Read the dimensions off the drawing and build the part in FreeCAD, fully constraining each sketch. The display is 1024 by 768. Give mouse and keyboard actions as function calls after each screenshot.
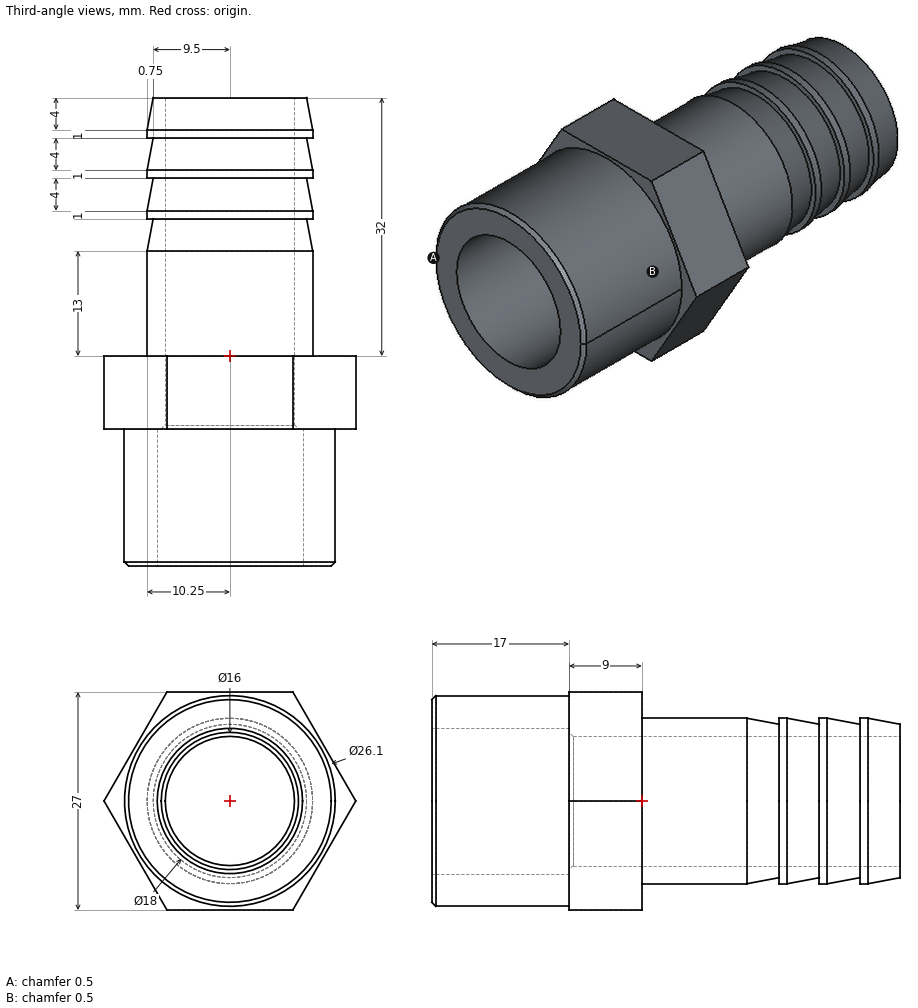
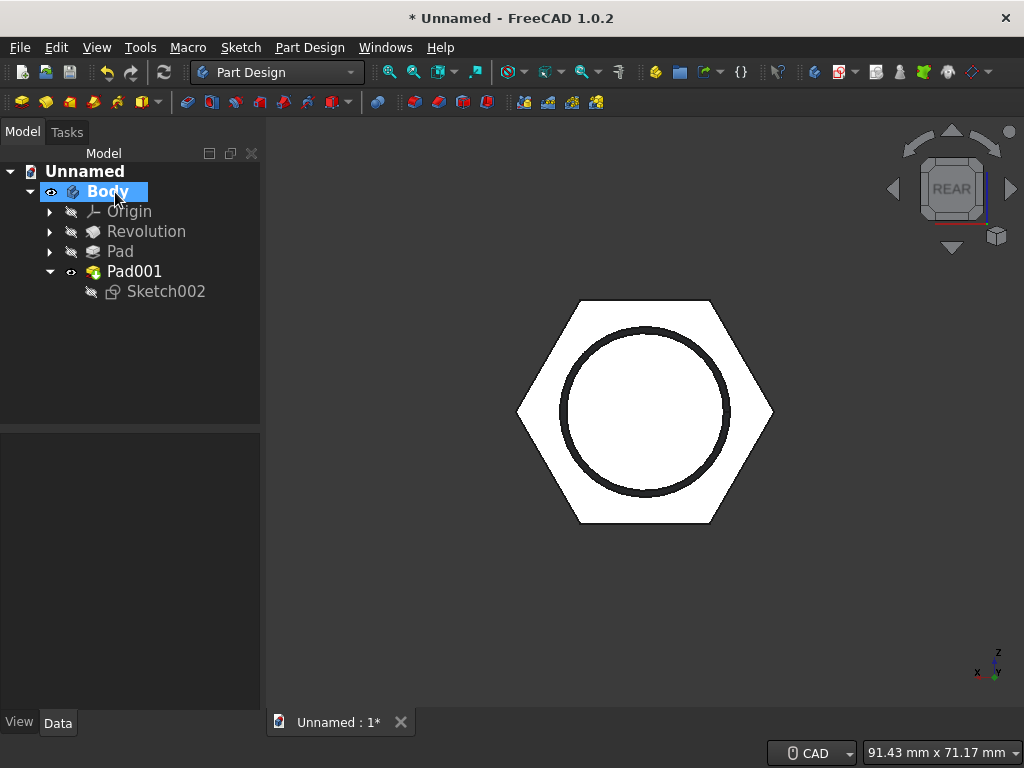
key(v)
key(f)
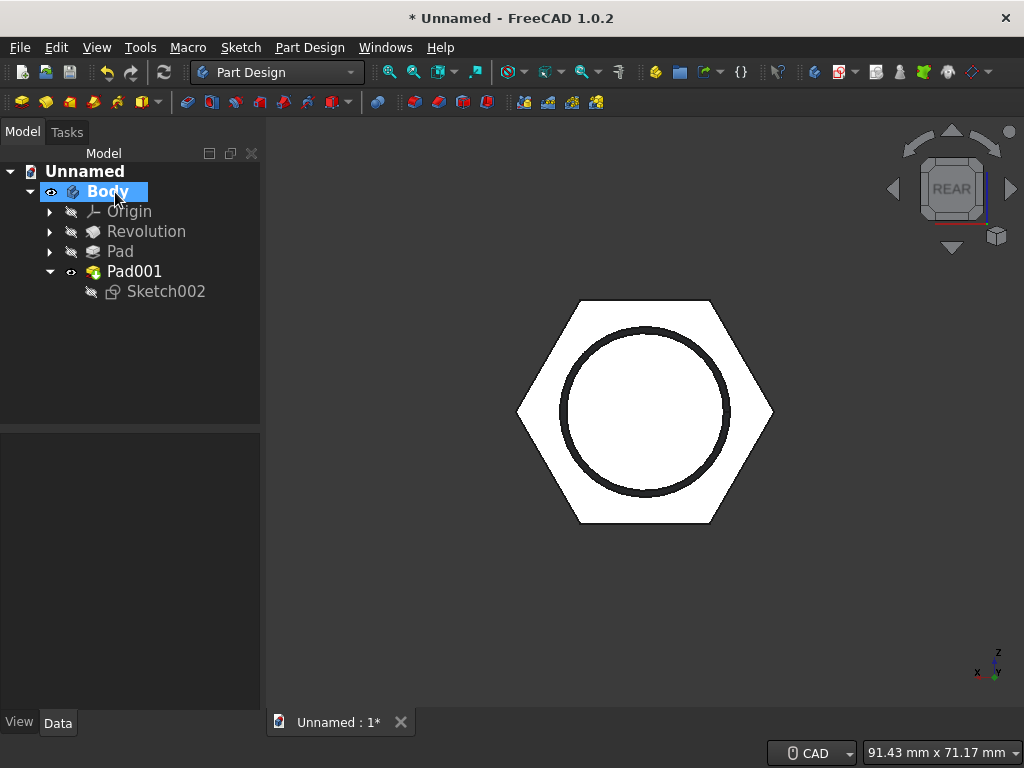
click(645, 411)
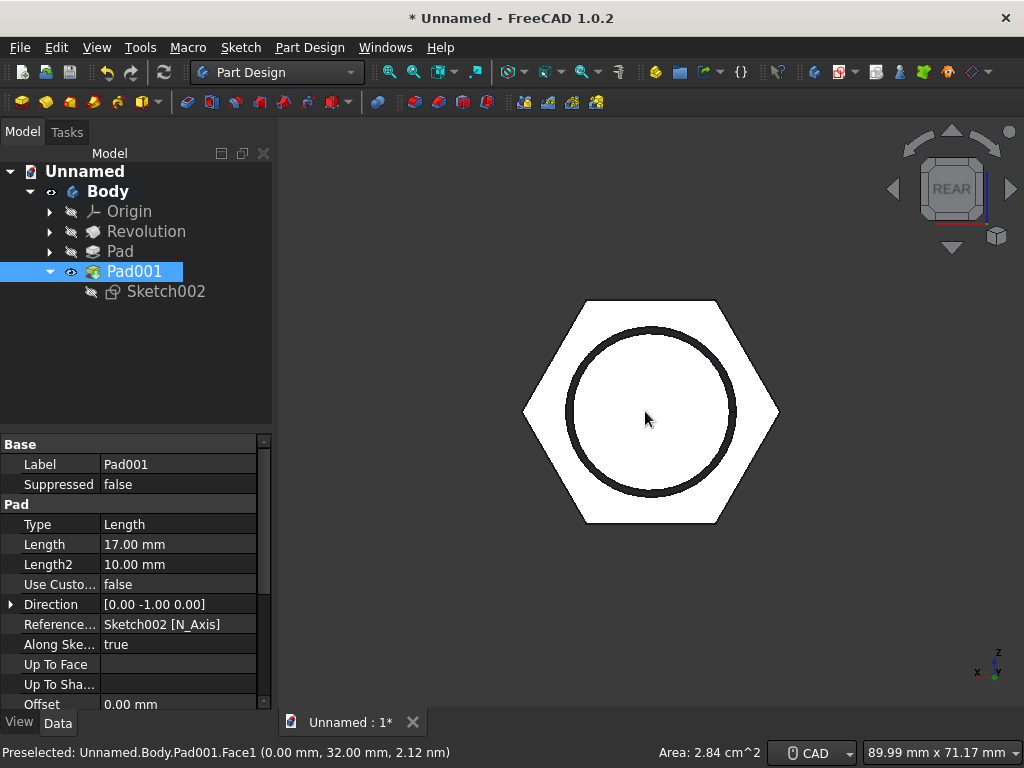
click(840, 72)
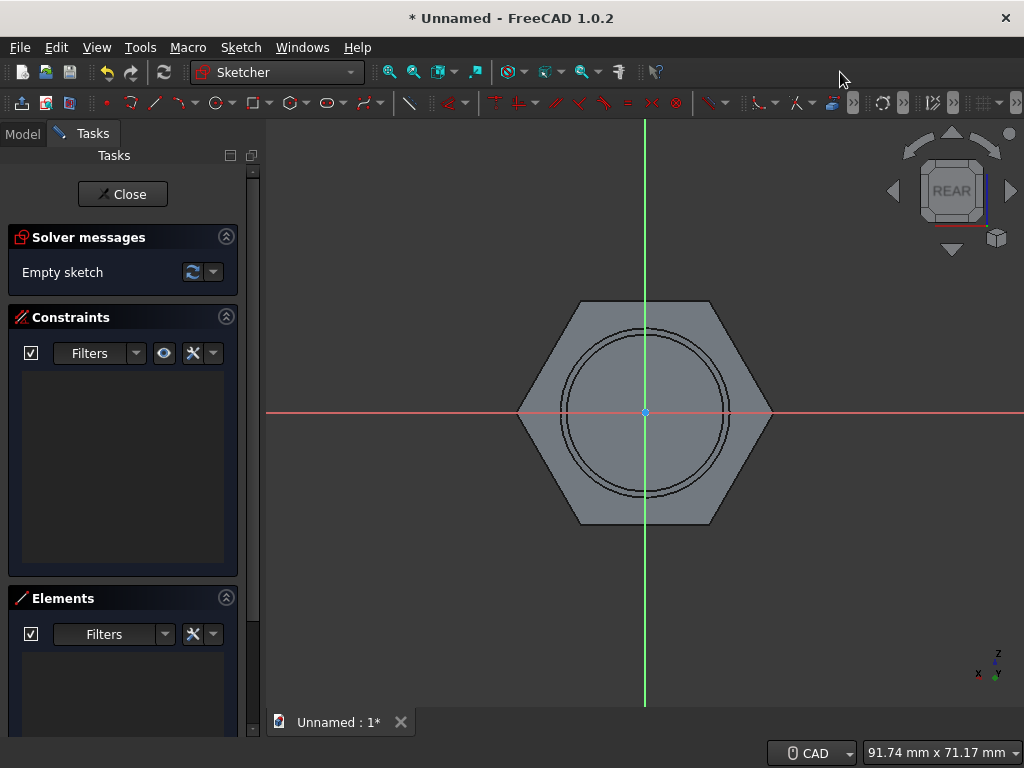
scroll(685, 413, up, 5)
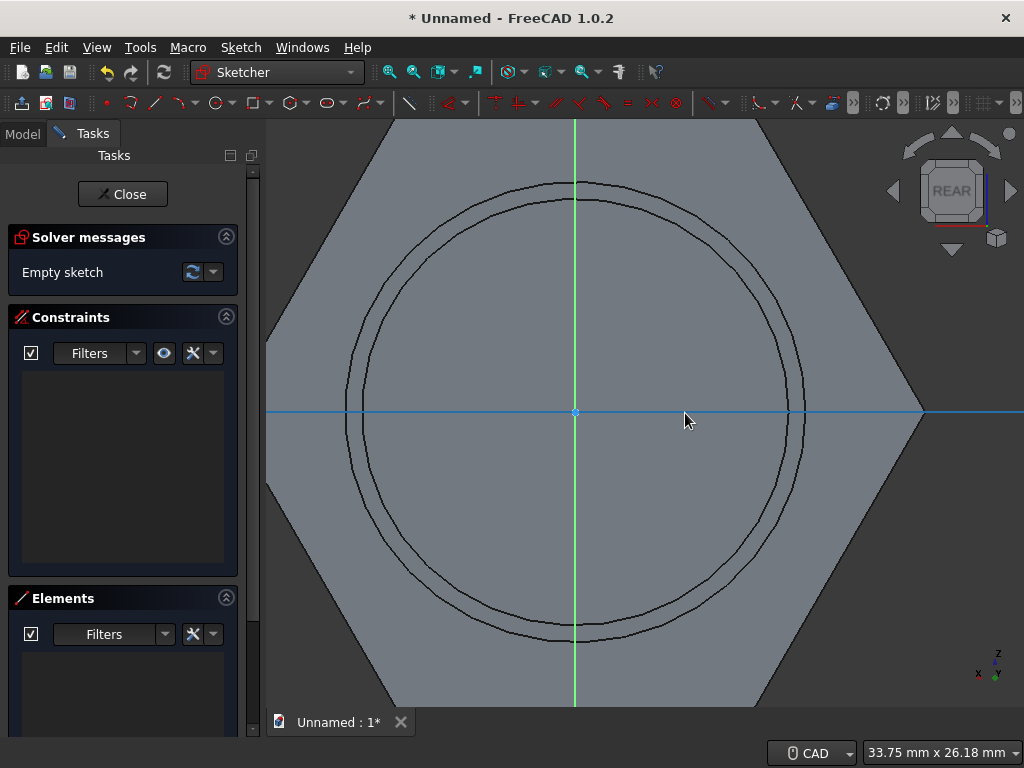
key(g)
key(c)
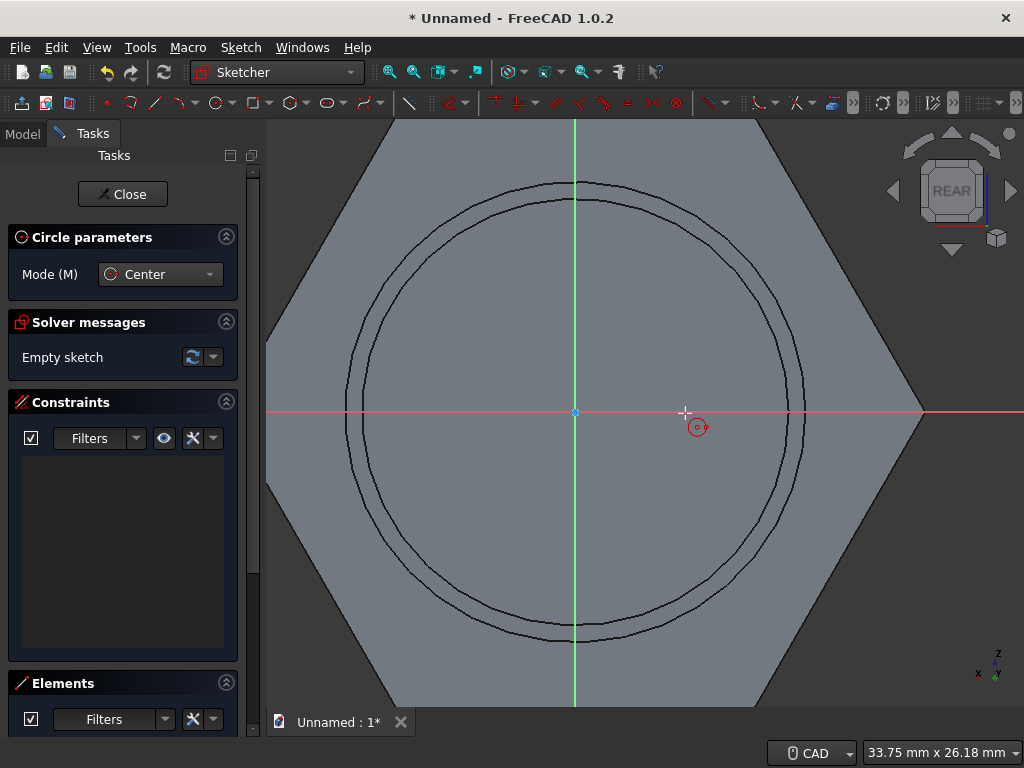
click(575, 412)
click(702, 285)
key(Escape)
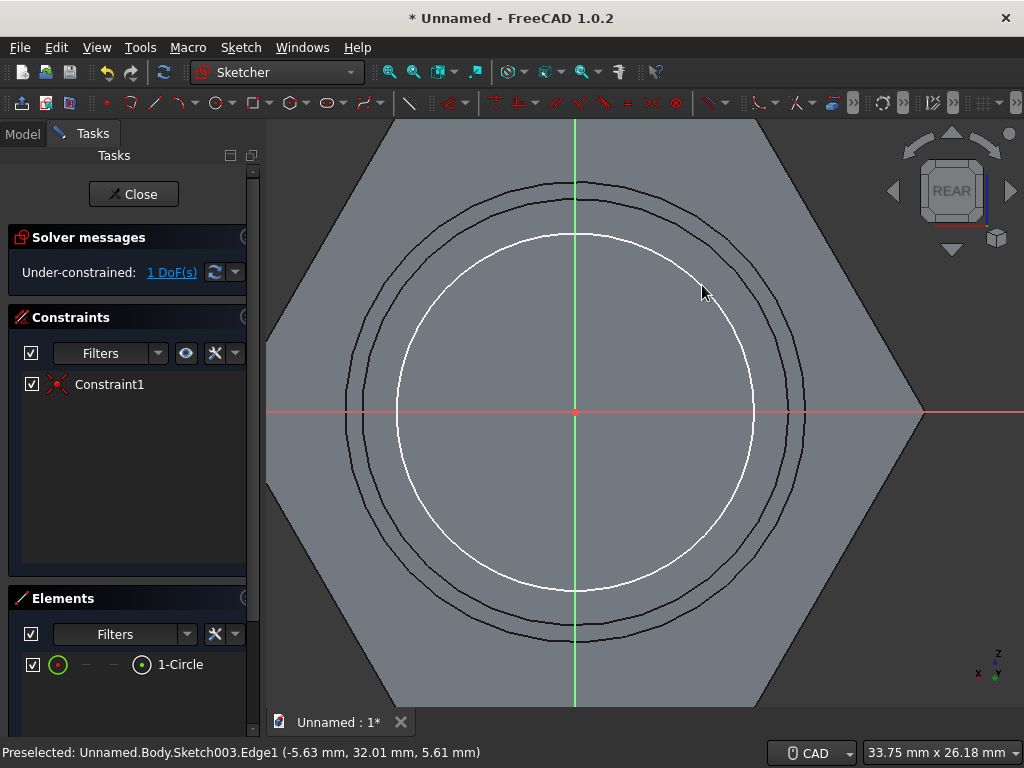
key(d)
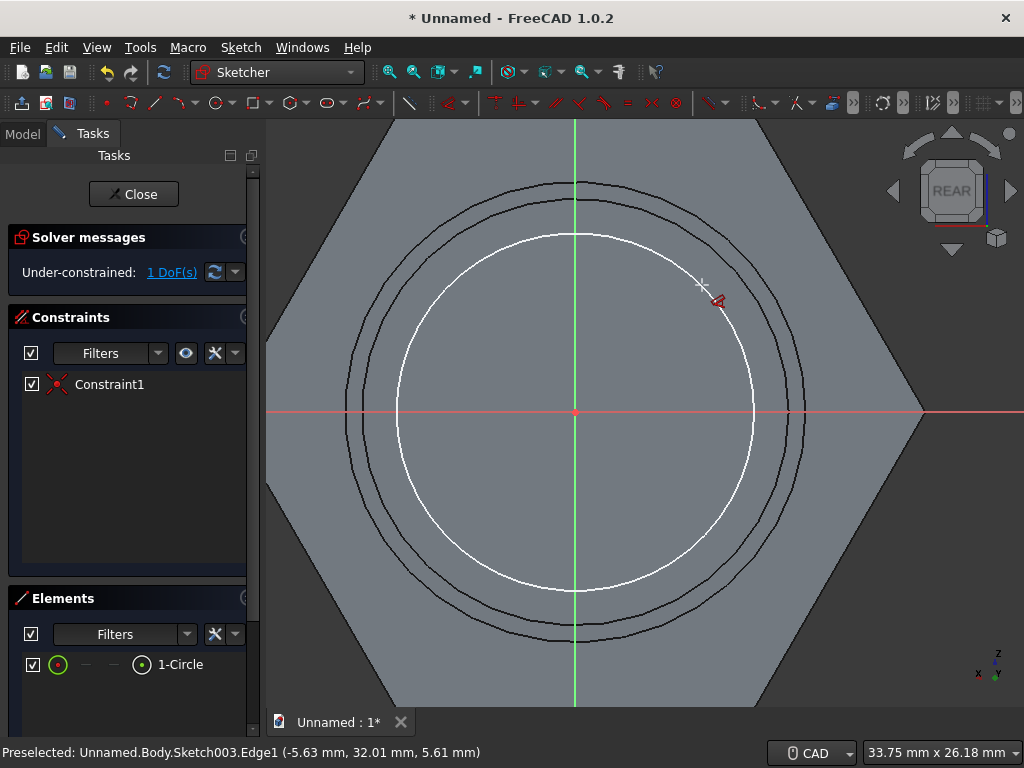
click(701, 285)
click(723, 262)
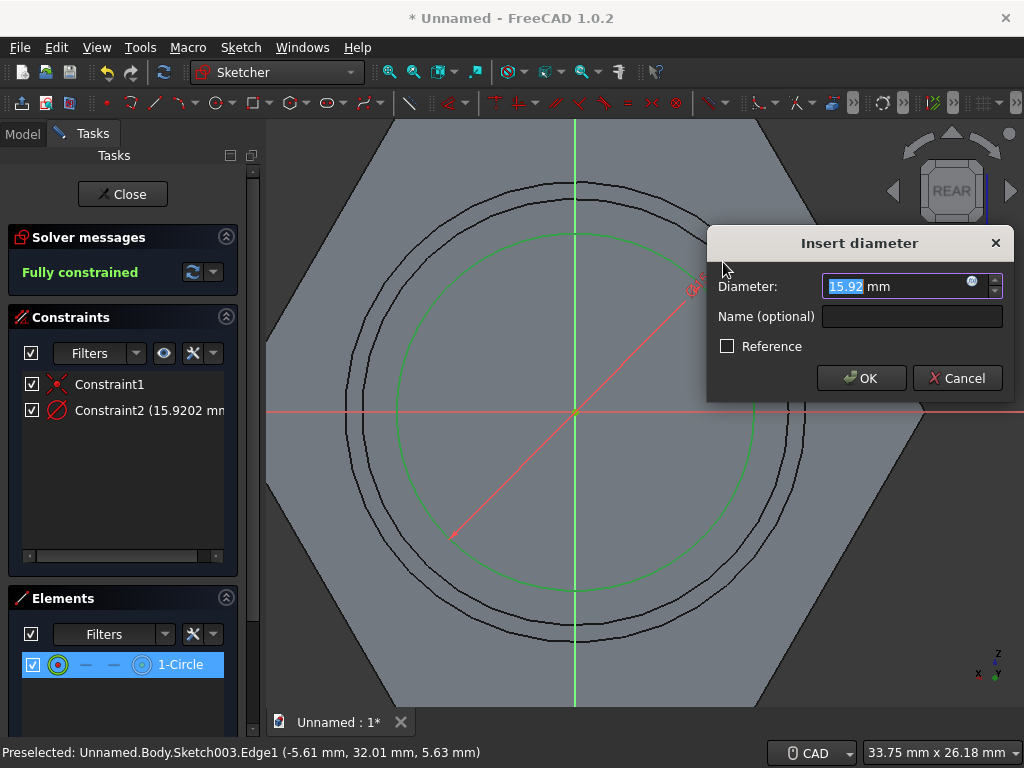
text(16)
key(Return)
key(Escape)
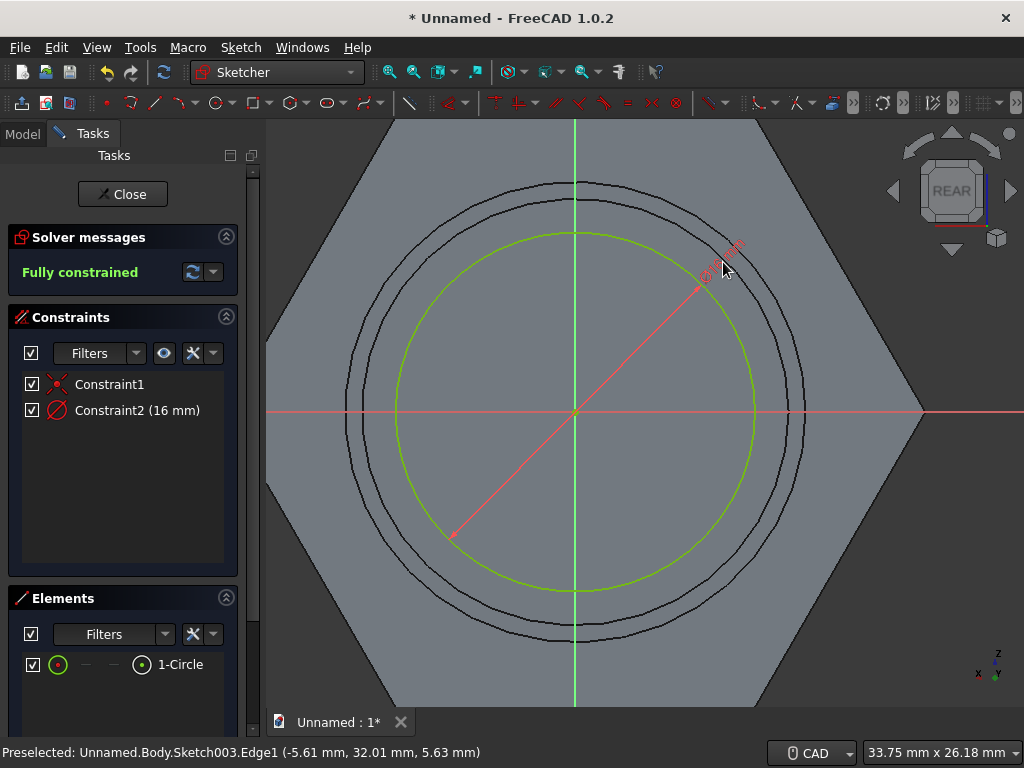
click(123, 194)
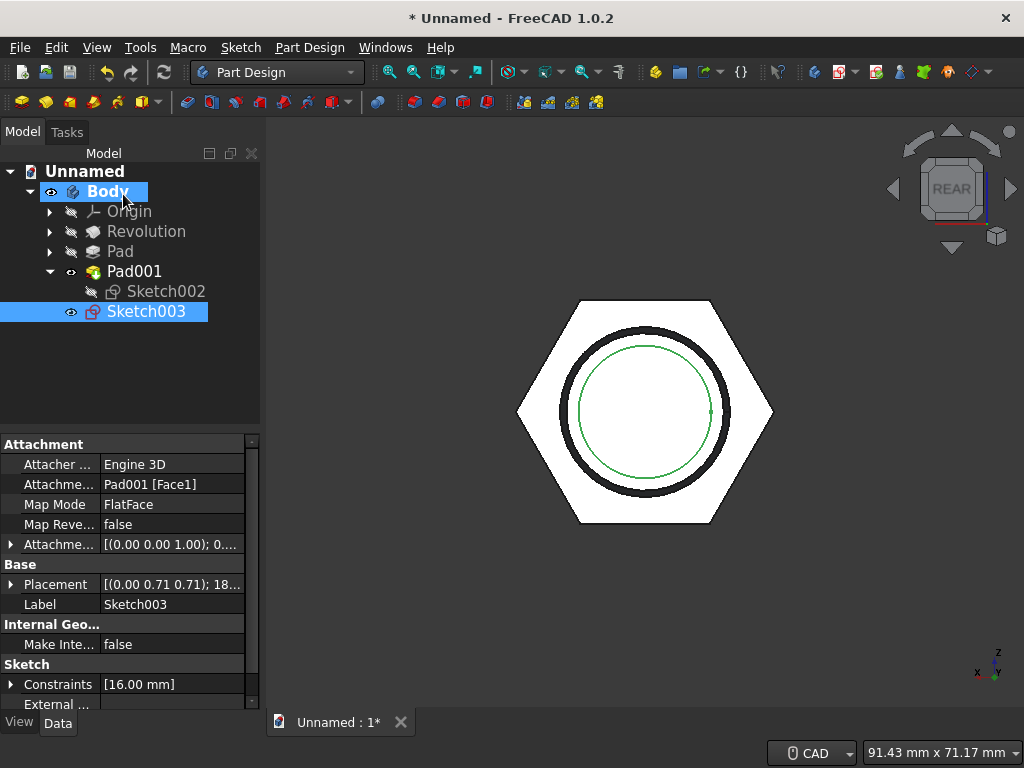
click(188, 102)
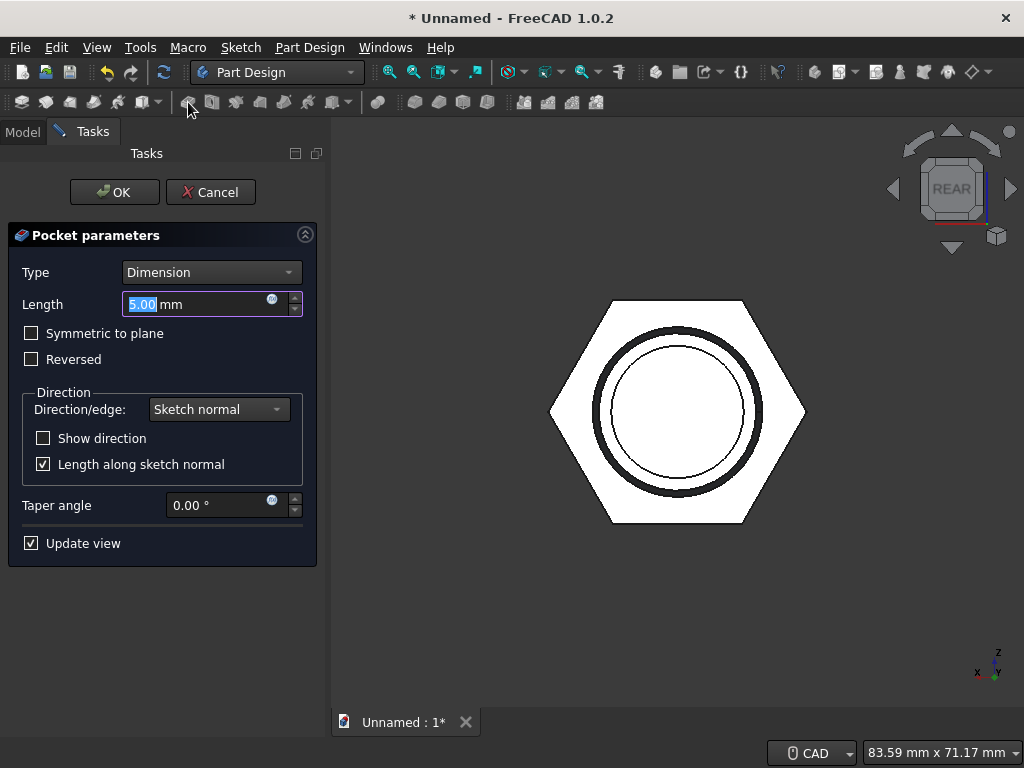
click(212, 272)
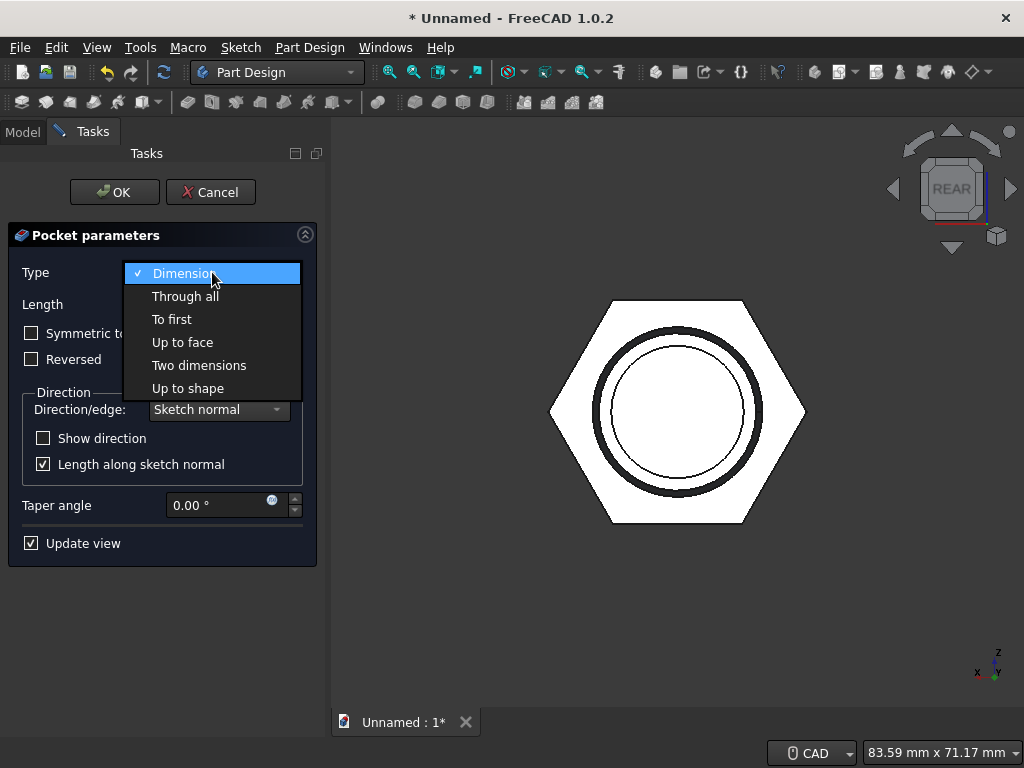
click(212, 320)